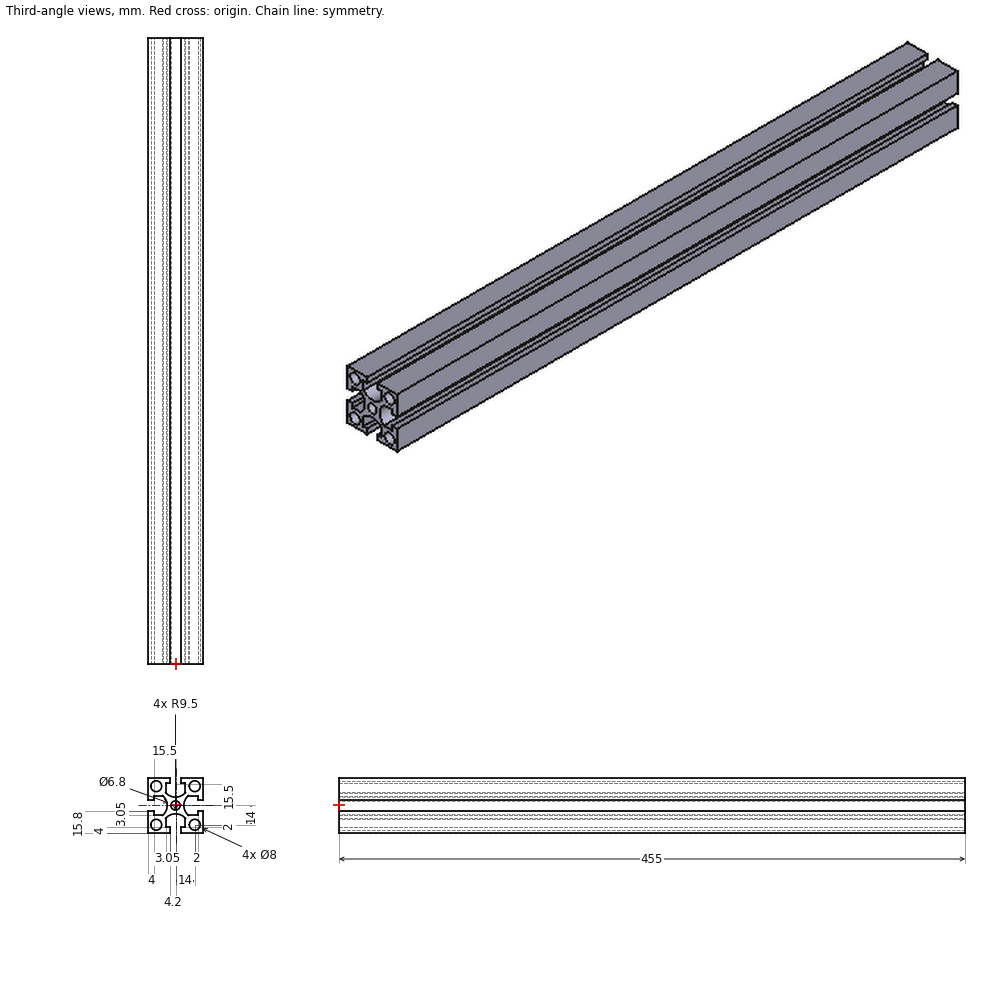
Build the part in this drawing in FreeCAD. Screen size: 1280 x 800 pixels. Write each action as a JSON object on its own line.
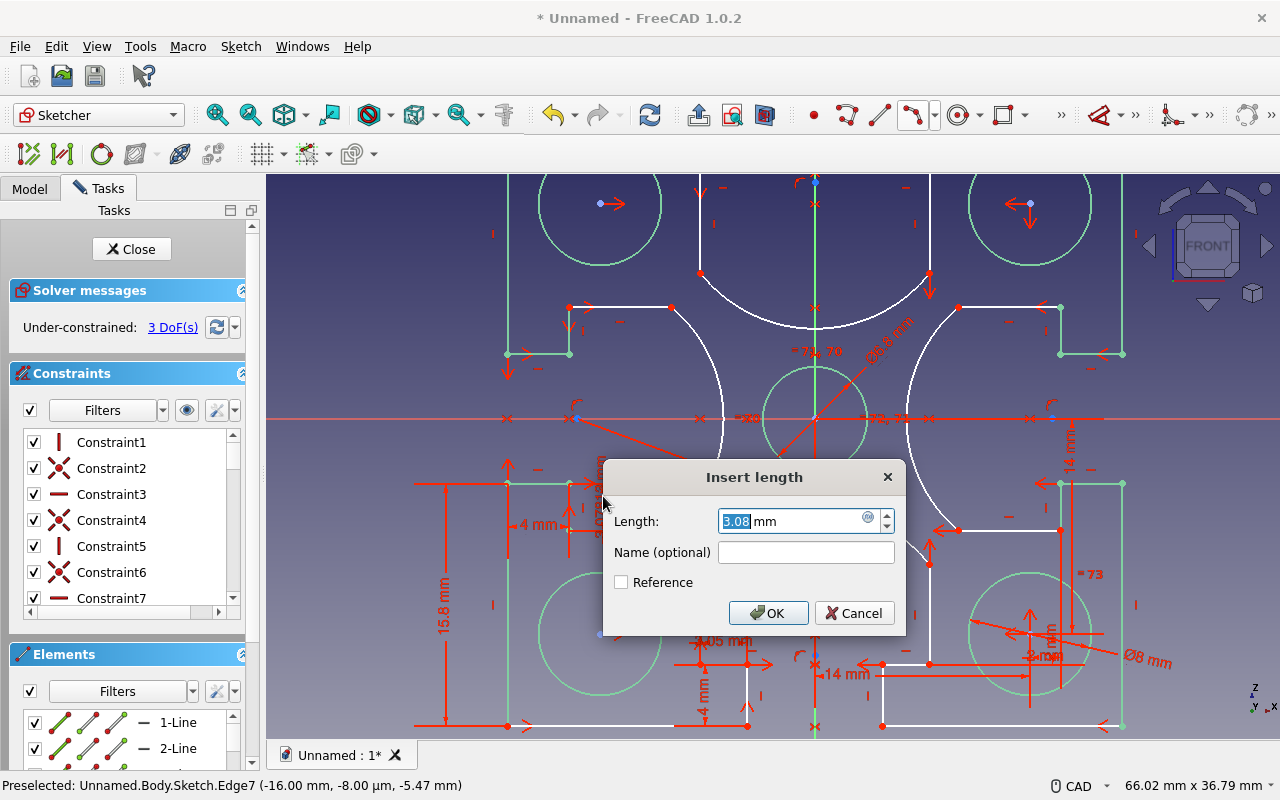
{"action": "type", "text": "3.05"}
{"action": "key", "text": "Return"}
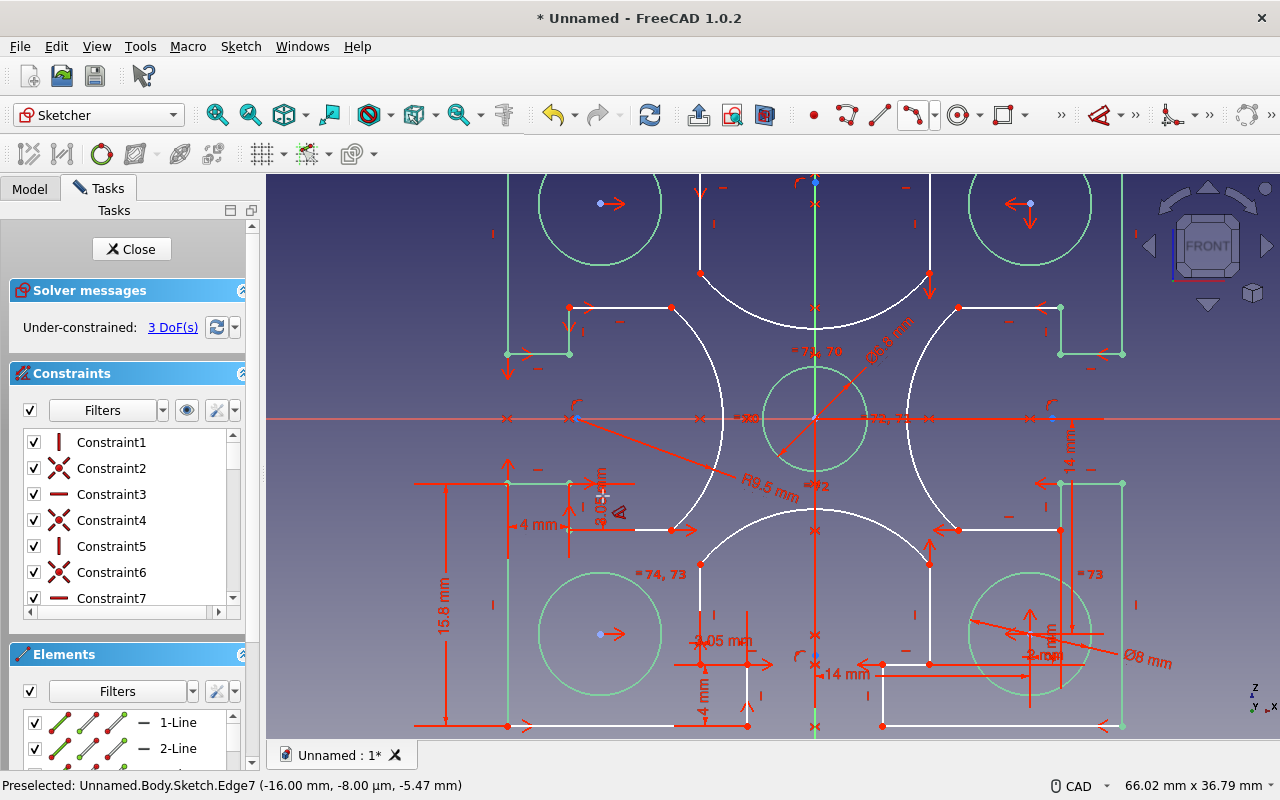
{"action": "left_click", "coordinate": [747, 665]}
{"action": "left_click", "coordinate": [781, 699]}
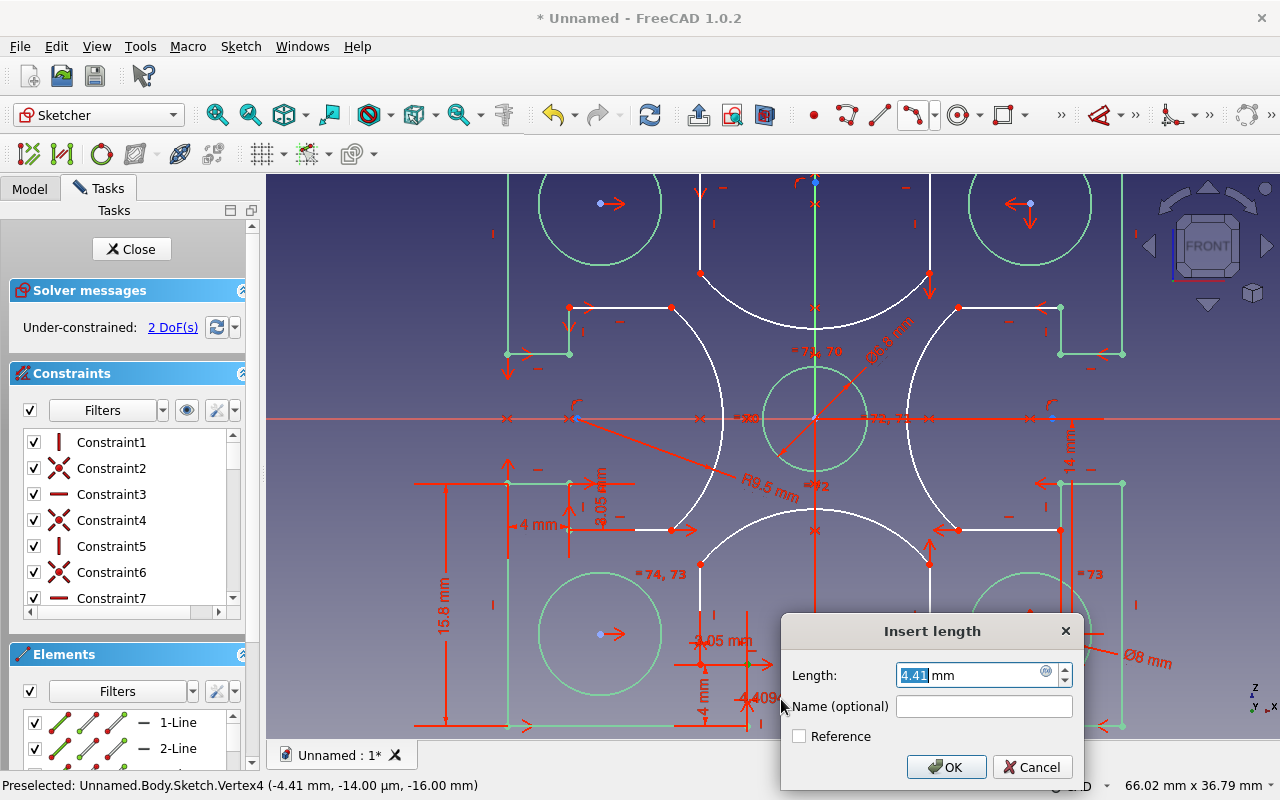
{"action": "type", "text": "4.2"}
{"action": "key", "text": "Return"}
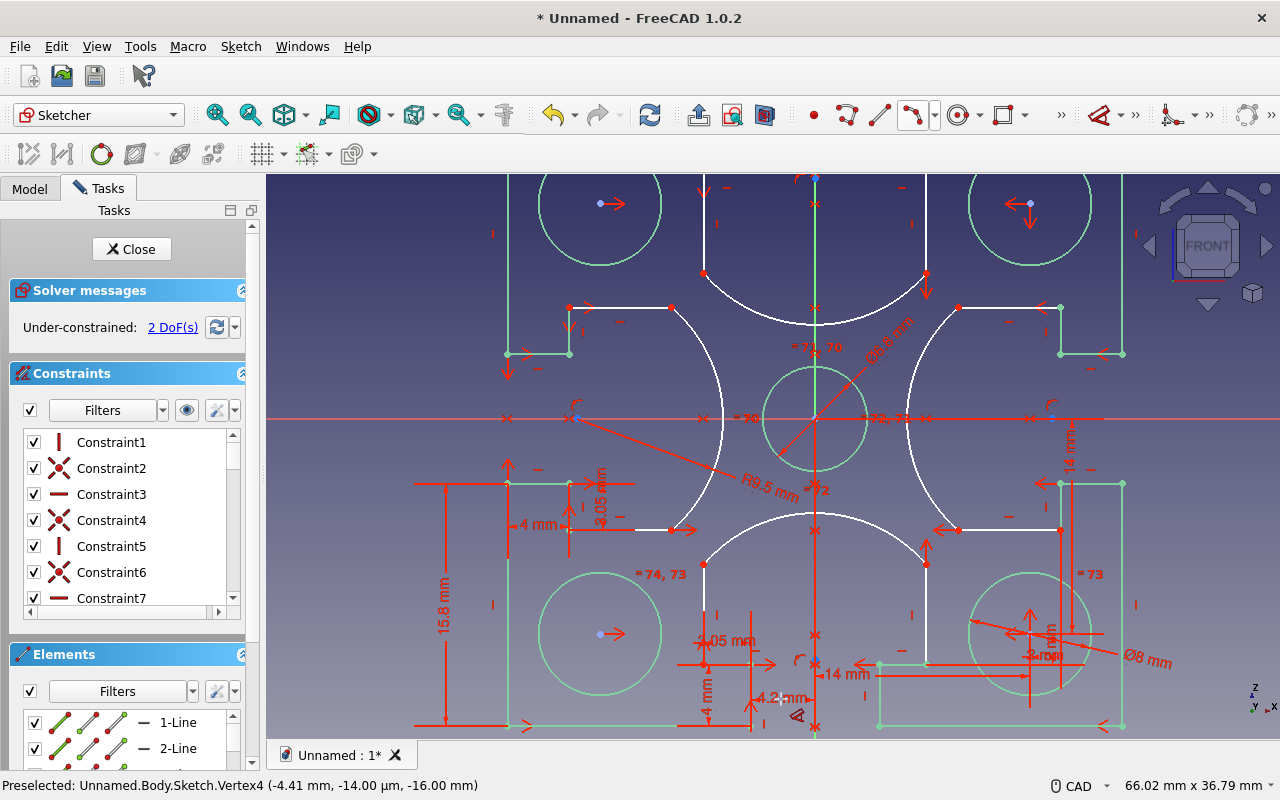
{"action": "left_click", "coordinate": [577, 419]}
{"action": "left_click", "coordinate": [696, 453]}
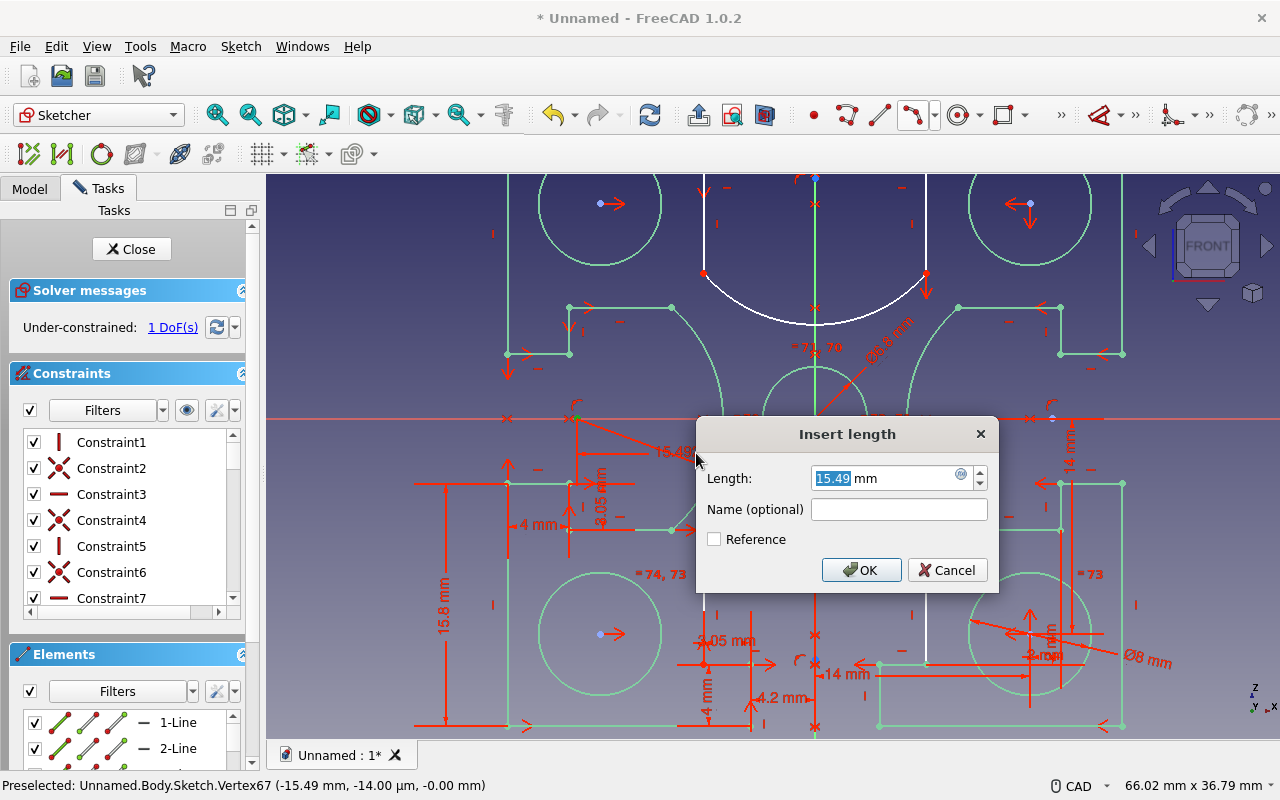
{"action": "type", "text": "15.5"}
{"action": "key", "text": "Return"}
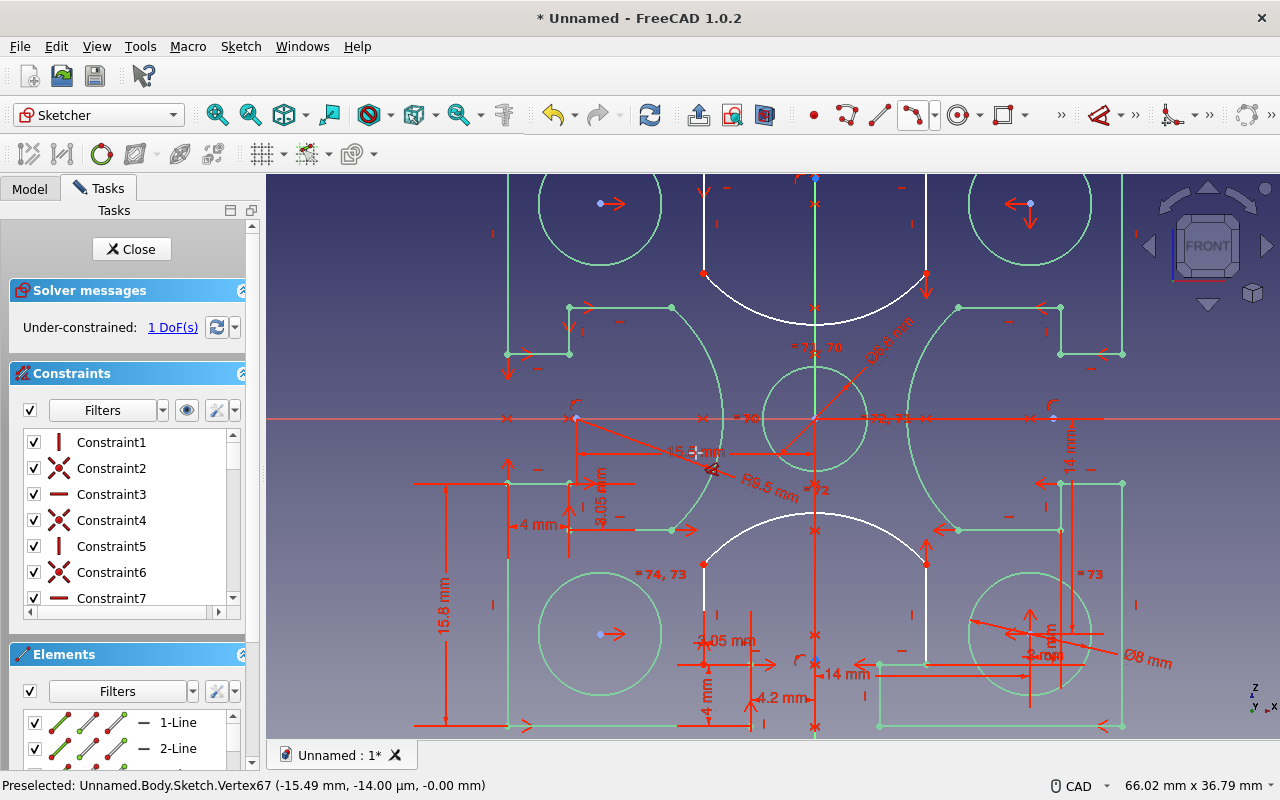
{"action": "scroll", "coordinate": [570, 502], "scroll_direction": "down", "scroll_amount": 3}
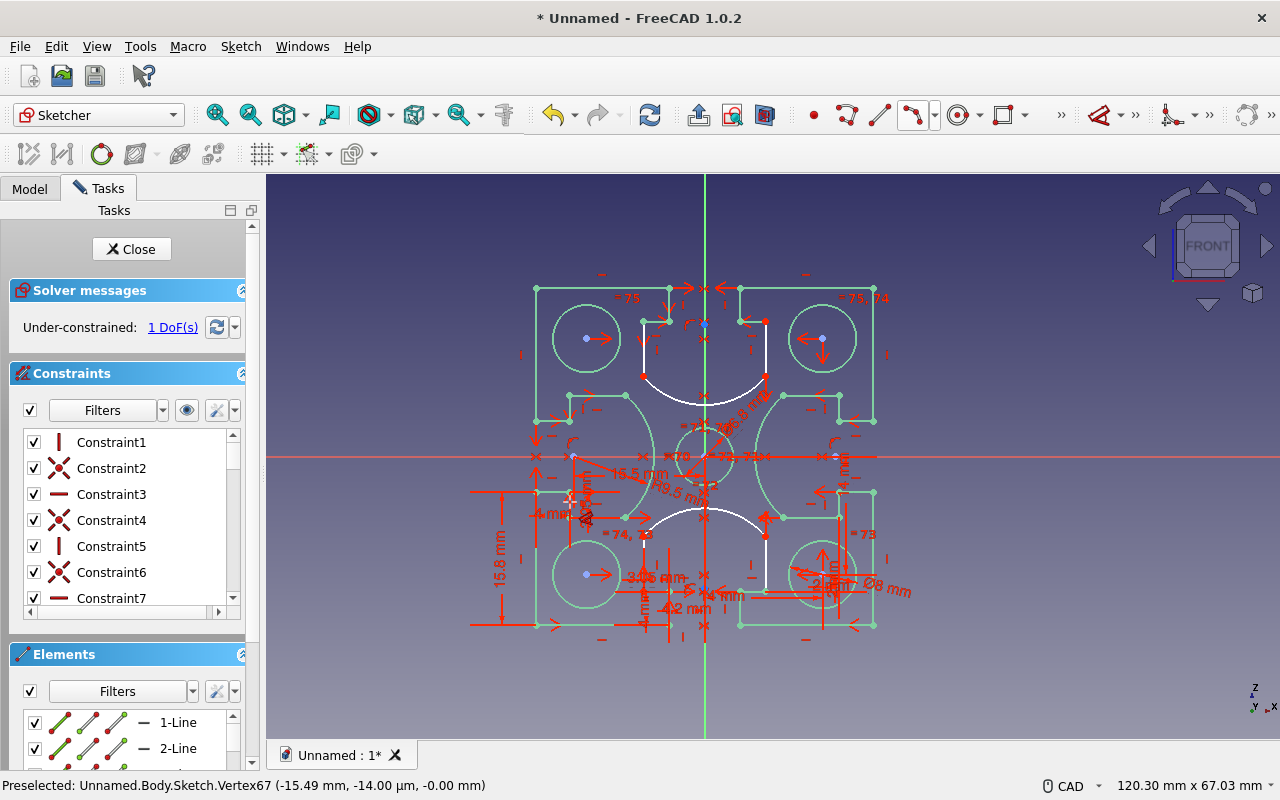
{"action": "left_click", "coordinate": [705, 325]}
{"action": "left_click", "coordinate": [739, 361]}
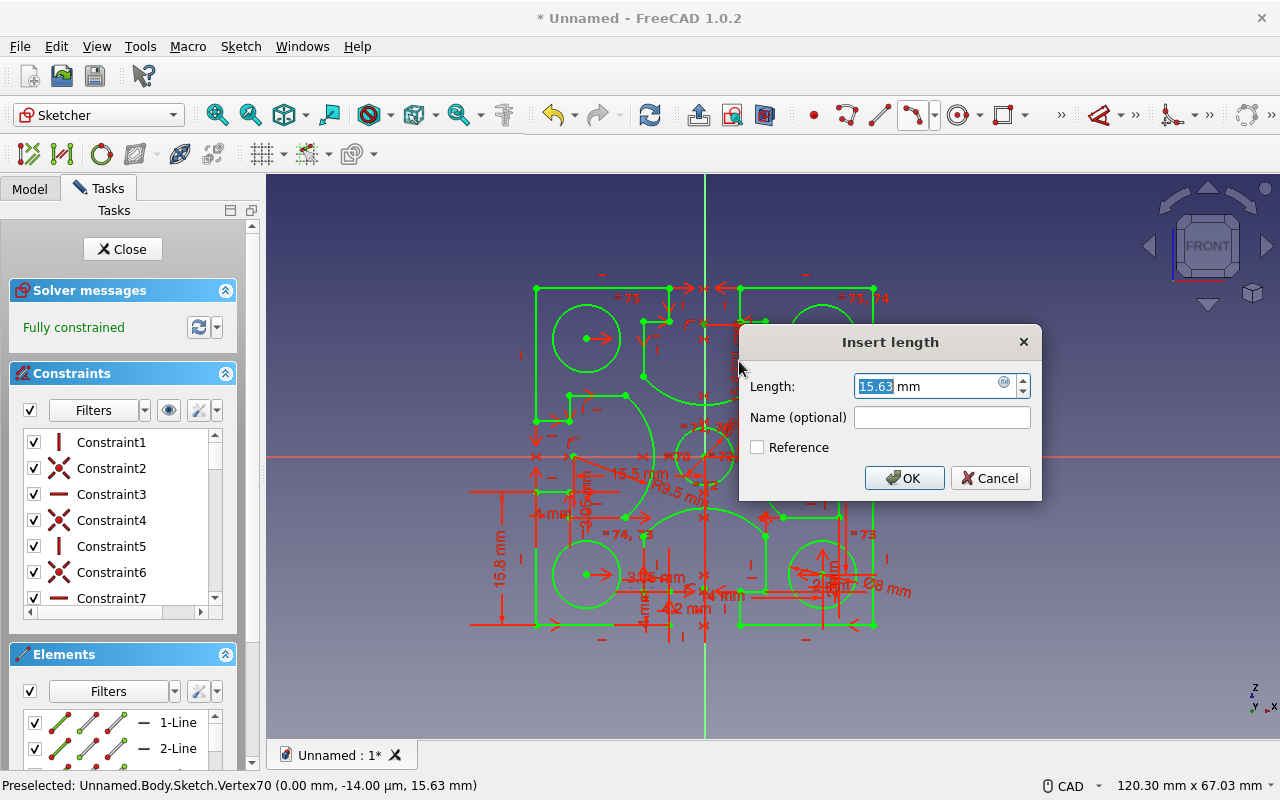
{"action": "type", "text": "15.5"}
{"action": "key", "text": "Return"}
{"action": "key", "text": "Escape"}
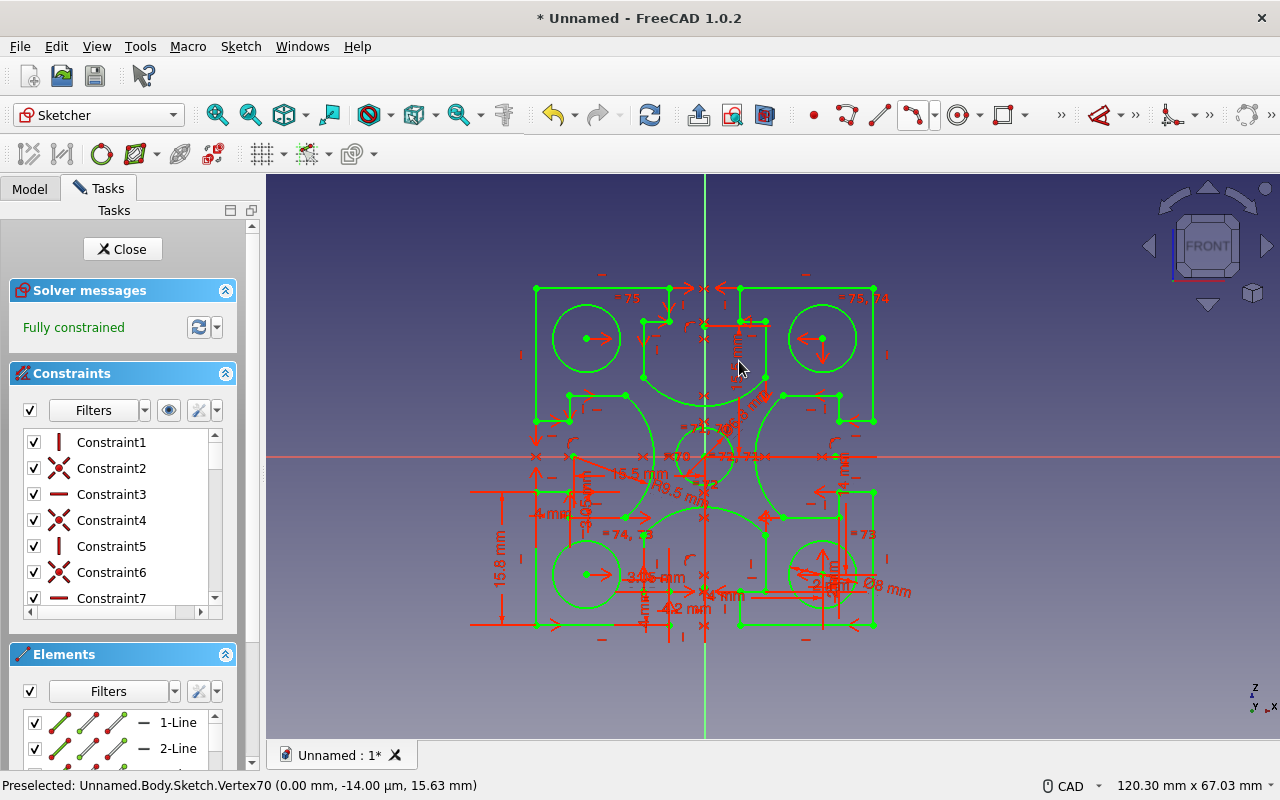
{"action": "left_click", "coordinate": [123, 249]}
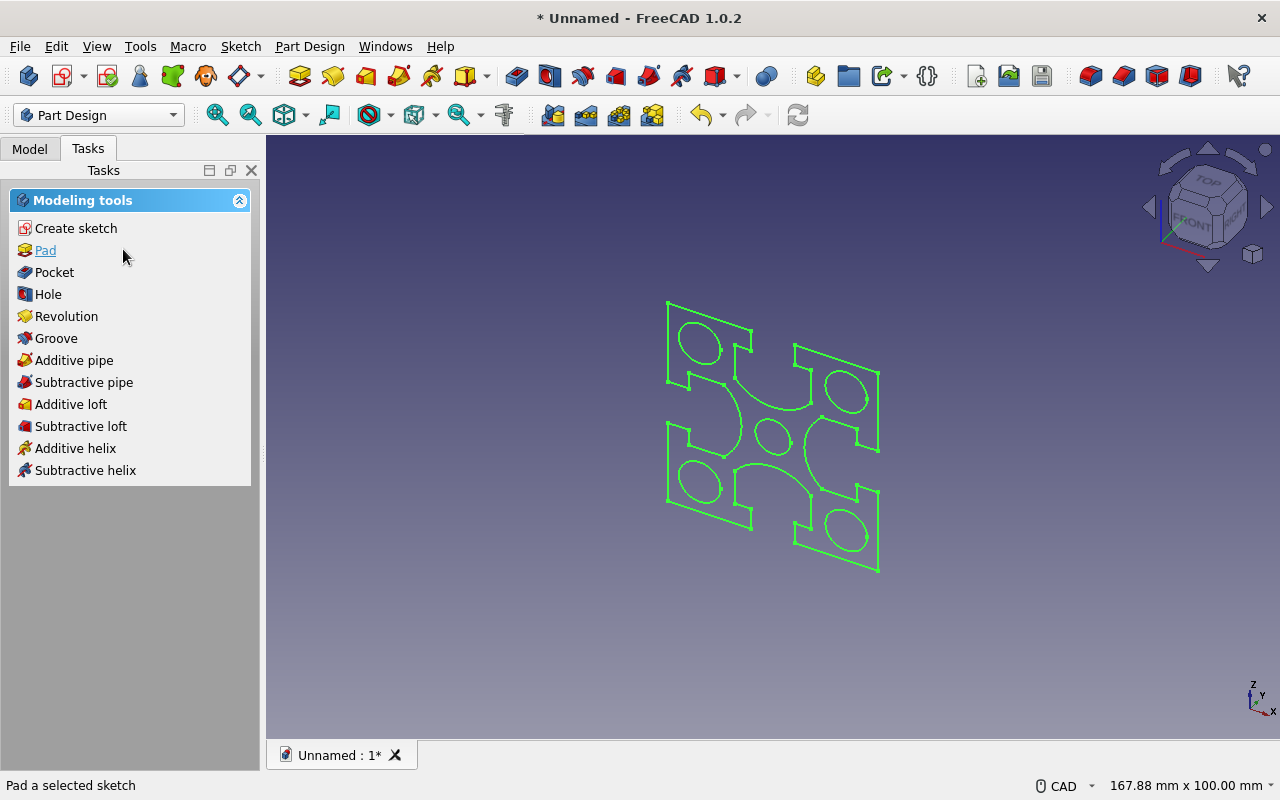
{"action": "left_click", "coordinate": [300, 76]}